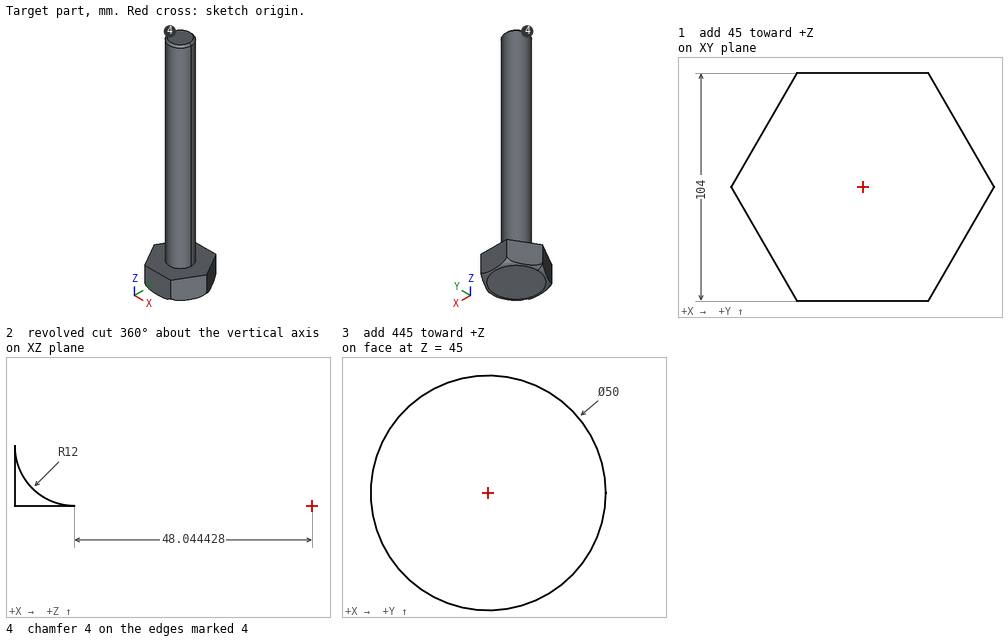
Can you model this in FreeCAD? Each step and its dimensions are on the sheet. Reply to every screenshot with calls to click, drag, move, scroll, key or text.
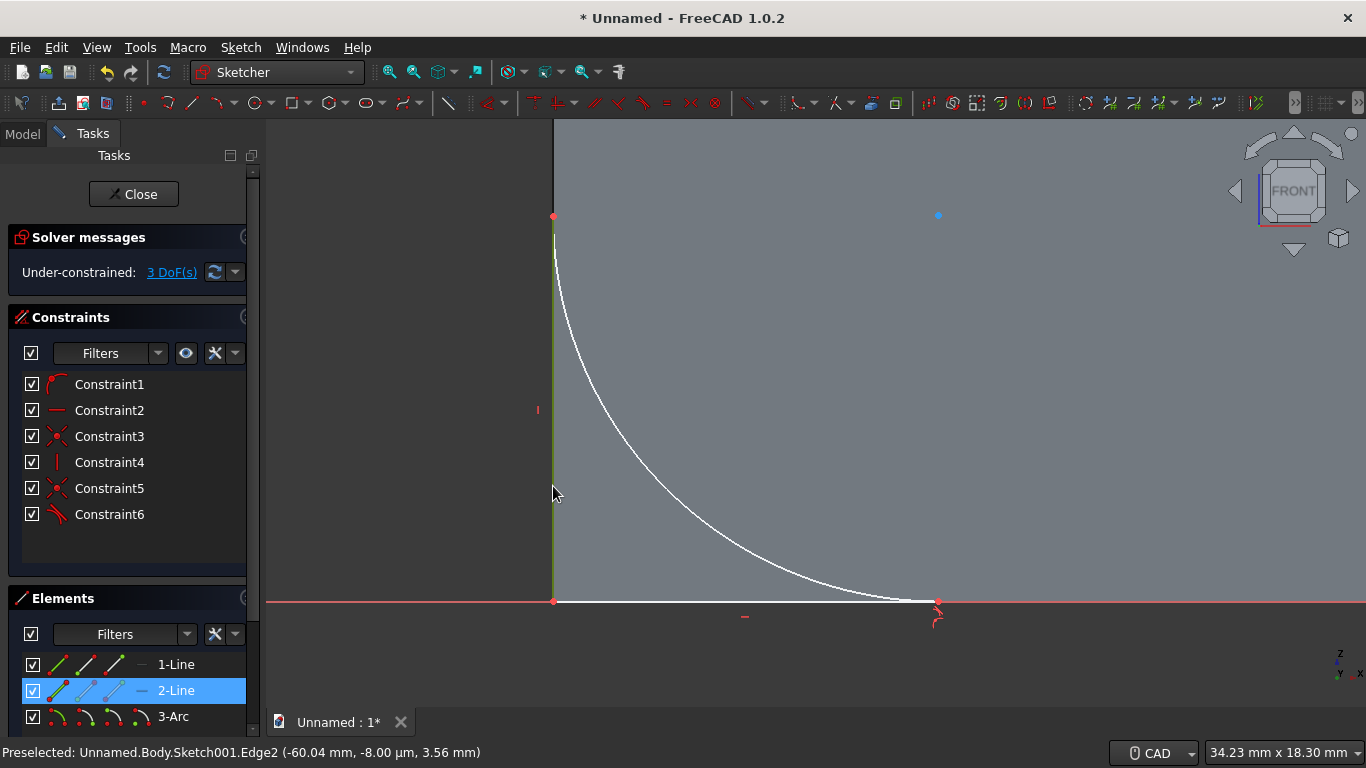
click(596, 392)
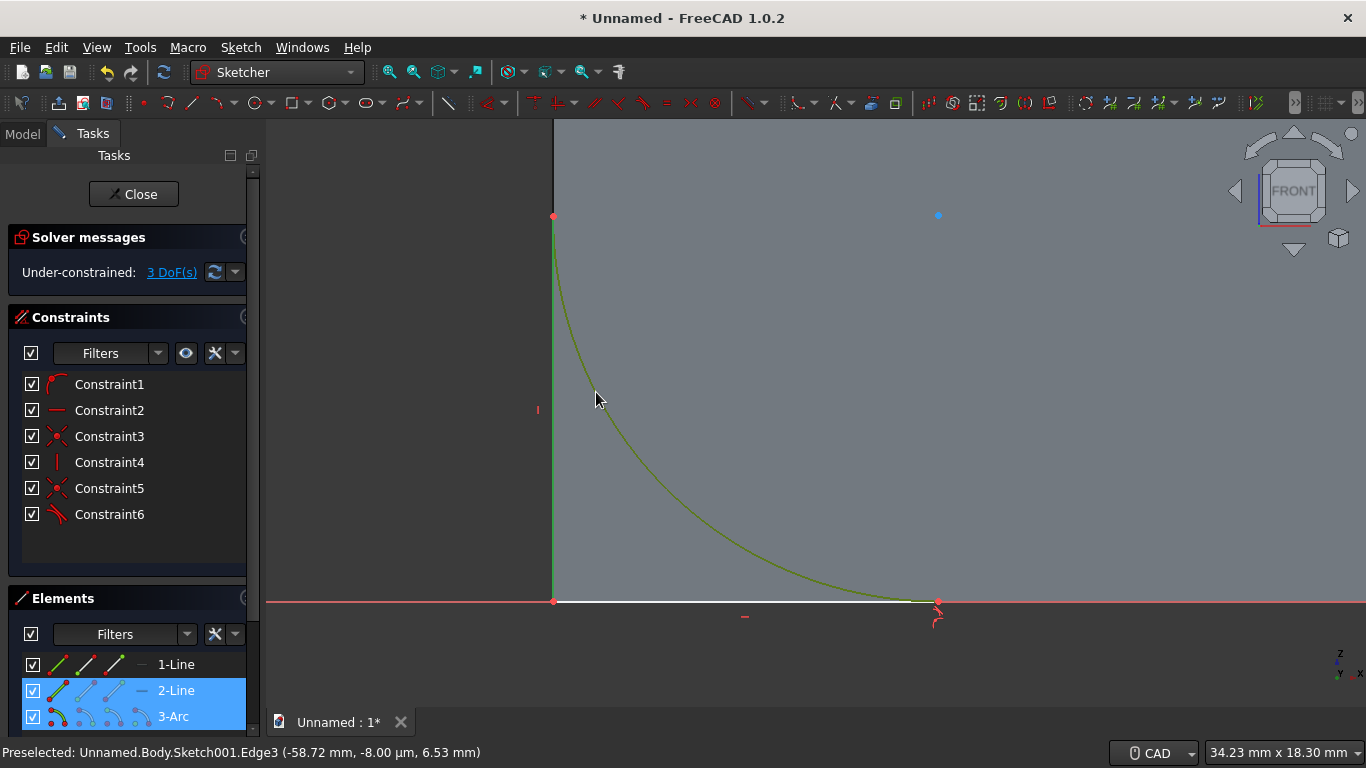
click(644, 104)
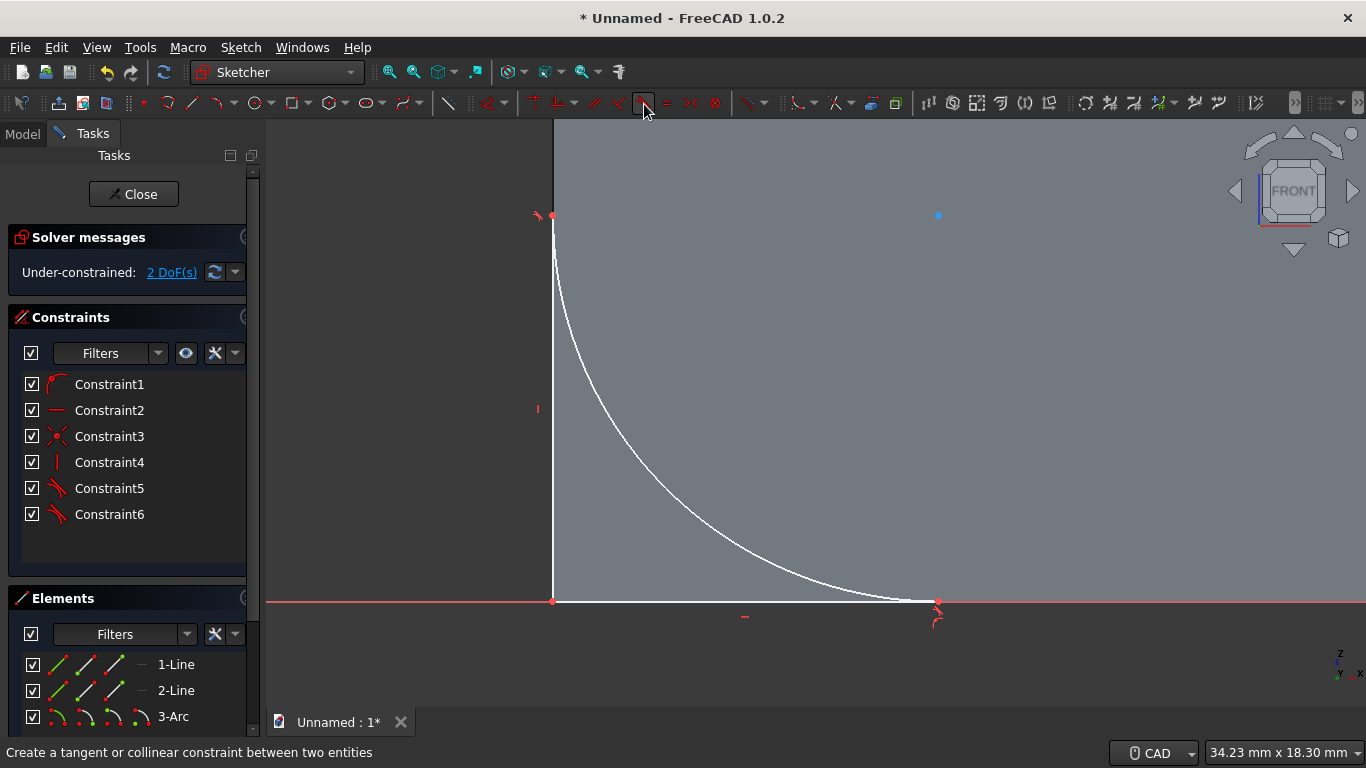
click(488, 104)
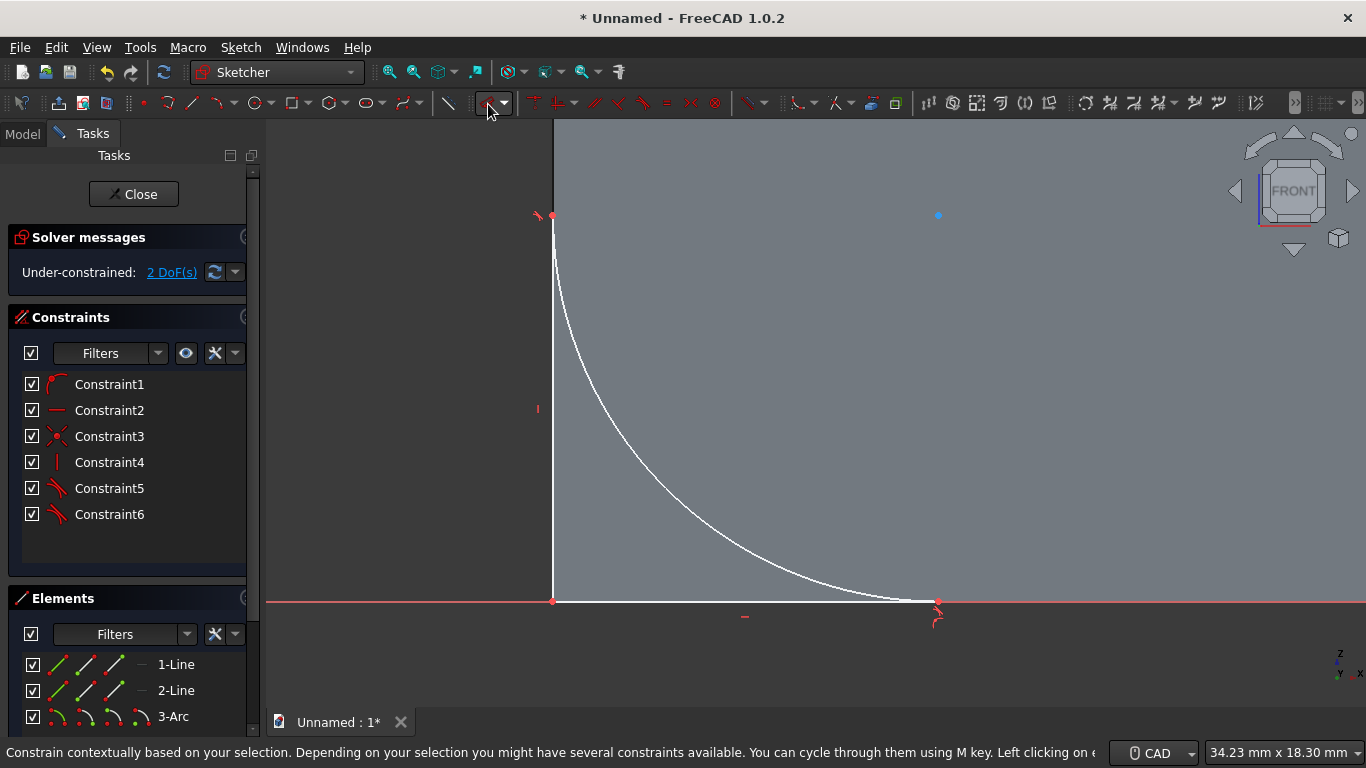
click(595, 391)
click(566, 406)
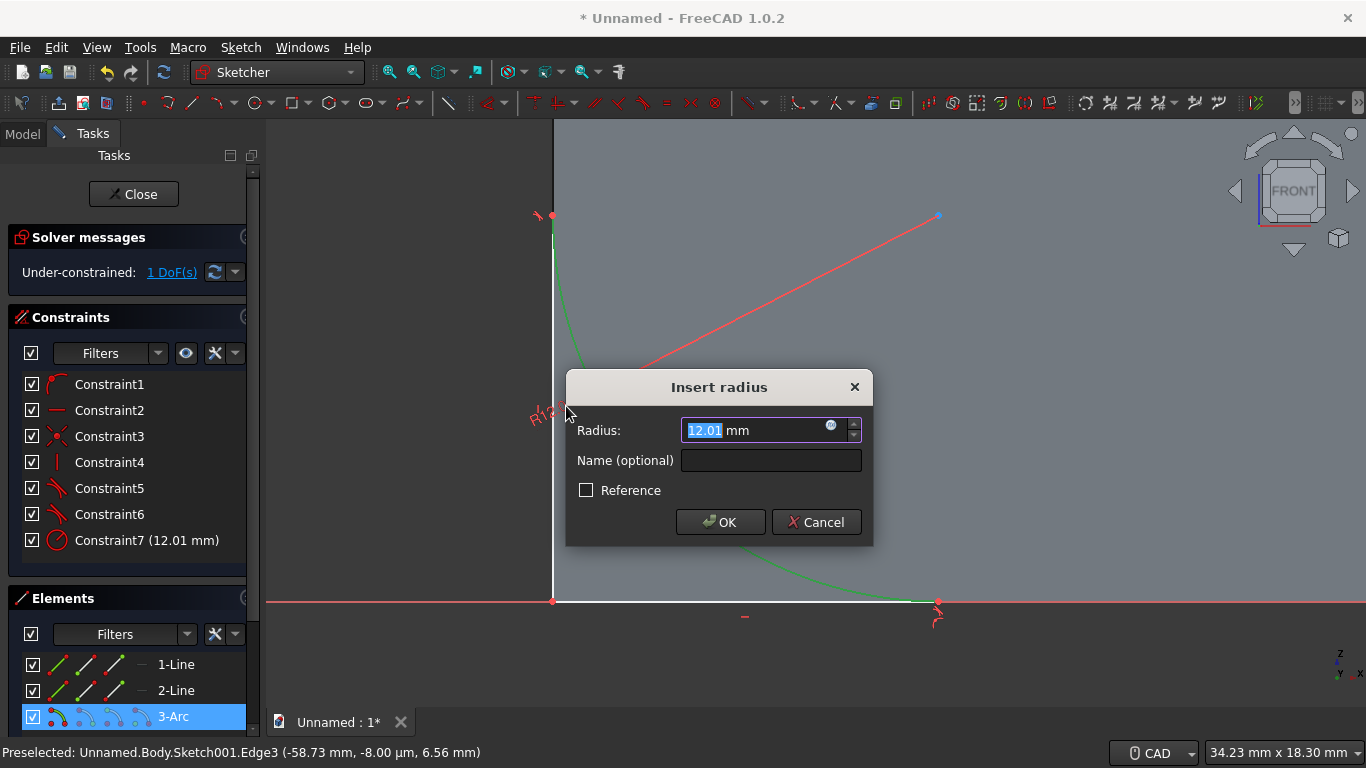
text(12)
key(Return)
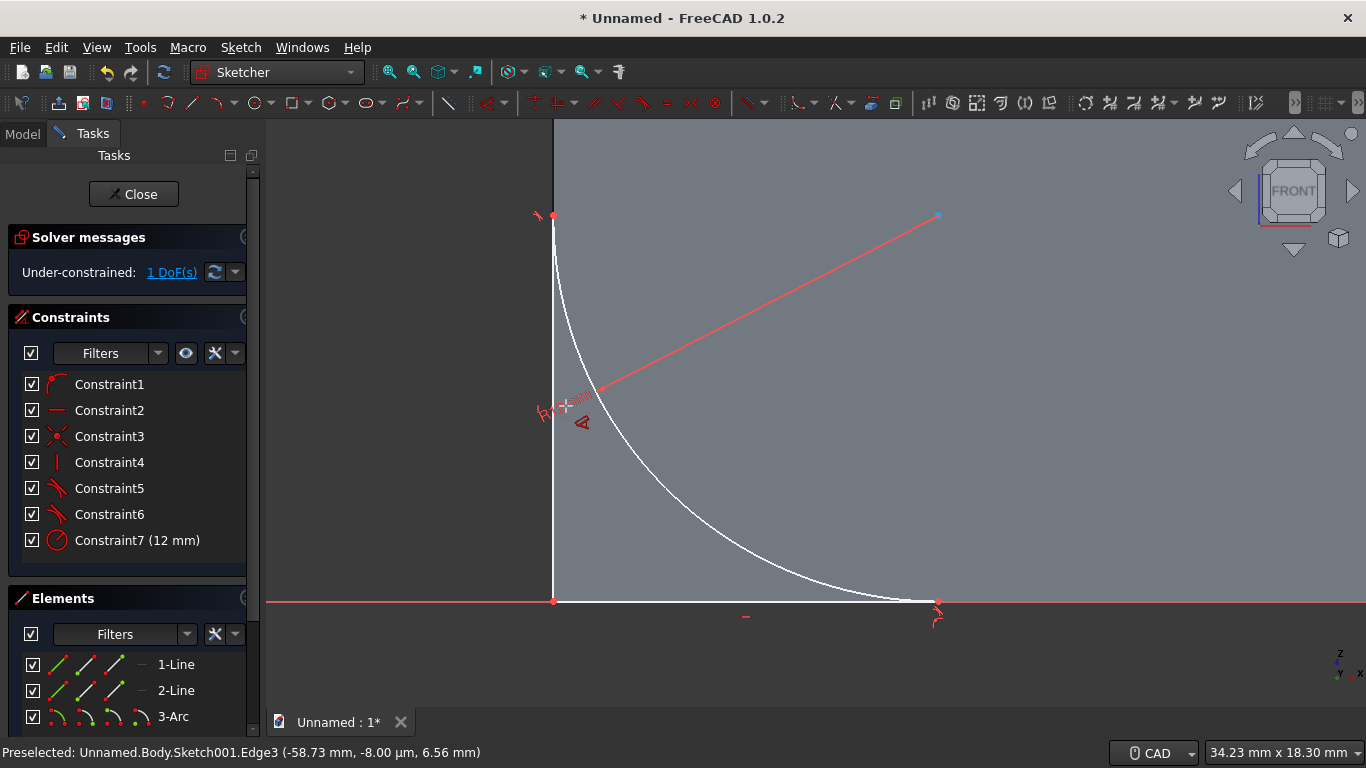
click(939, 602)
click(1070, 636)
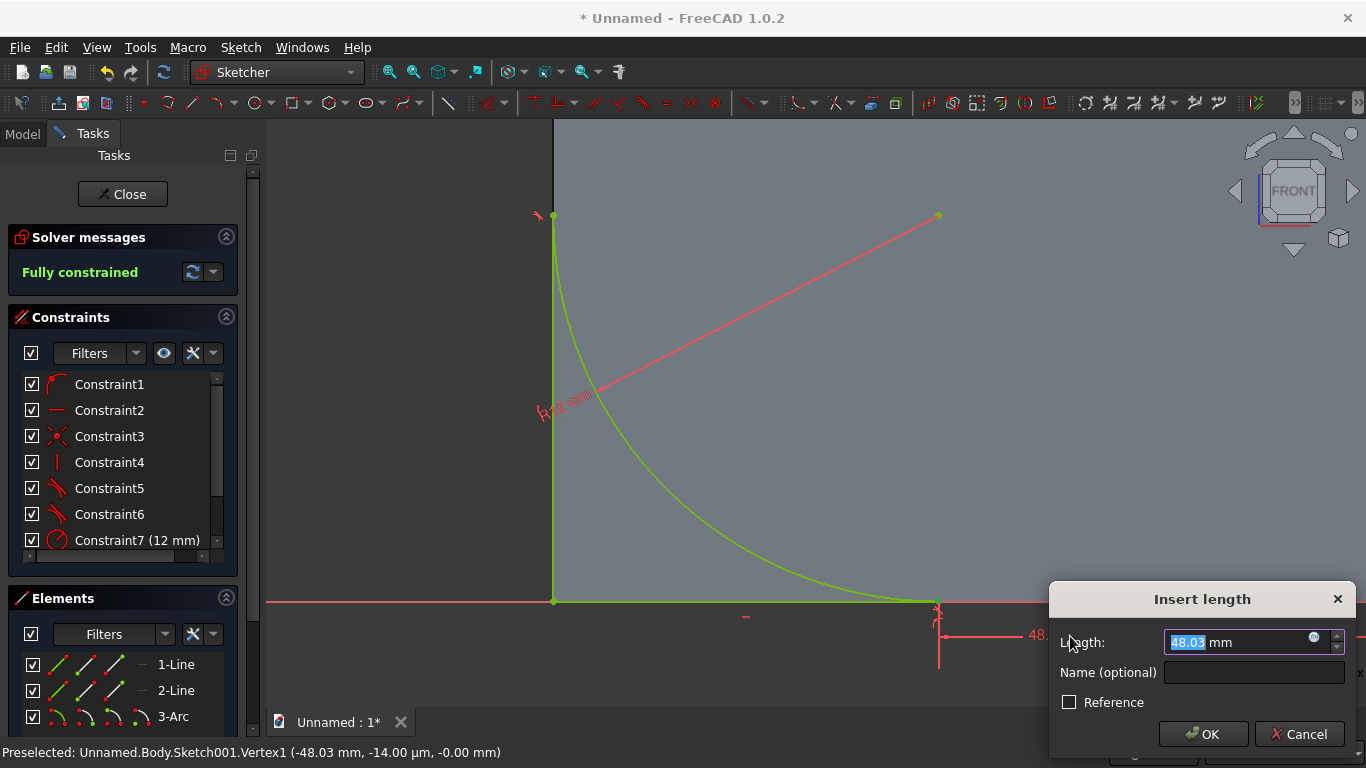
text(48.044428)
key(Return)
key(Escape)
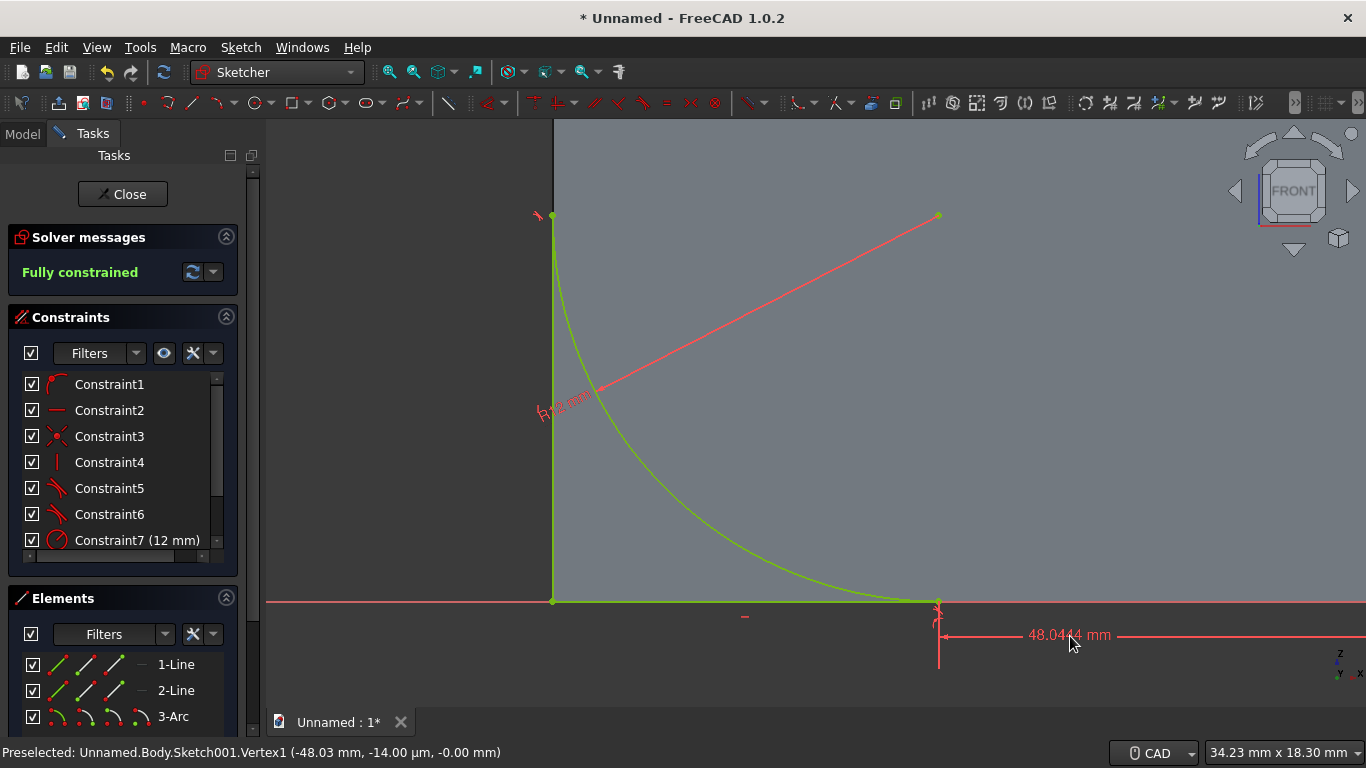
click(123, 194)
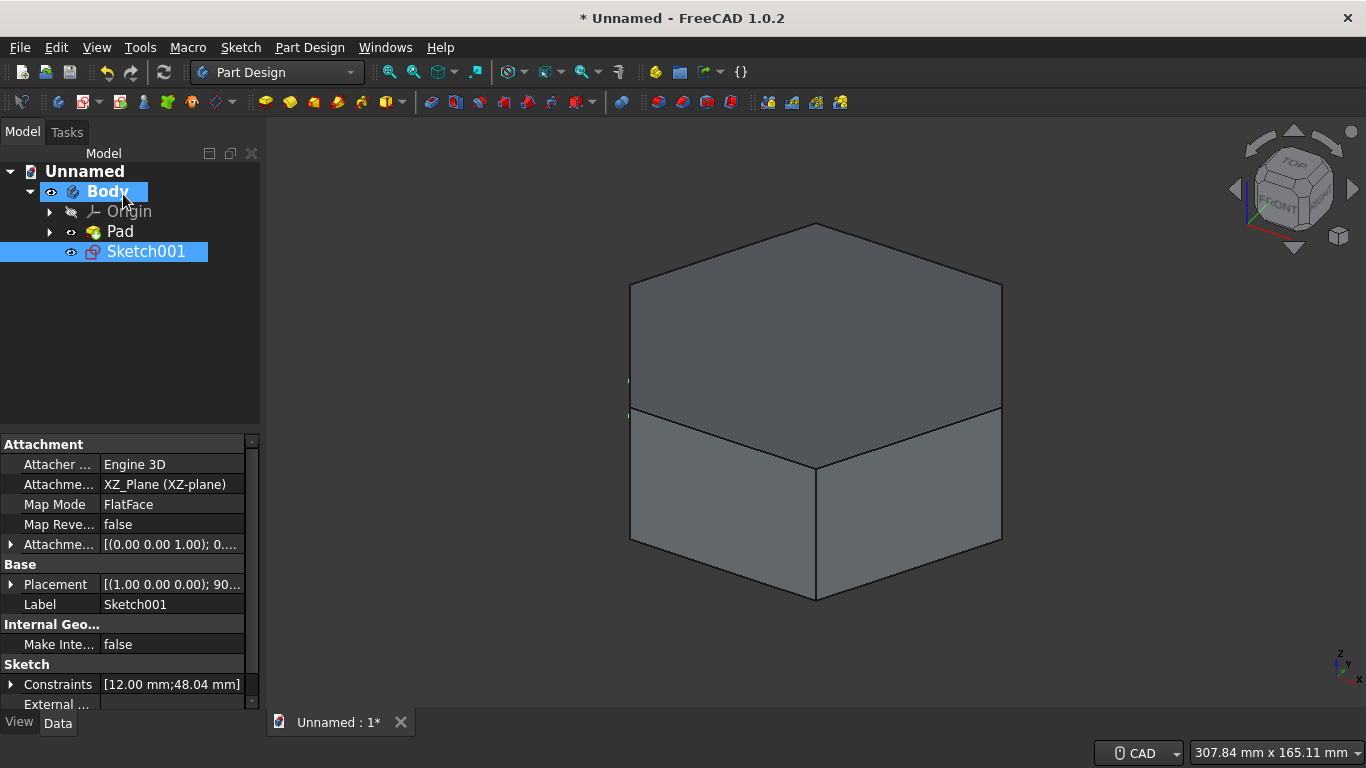
click(480, 102)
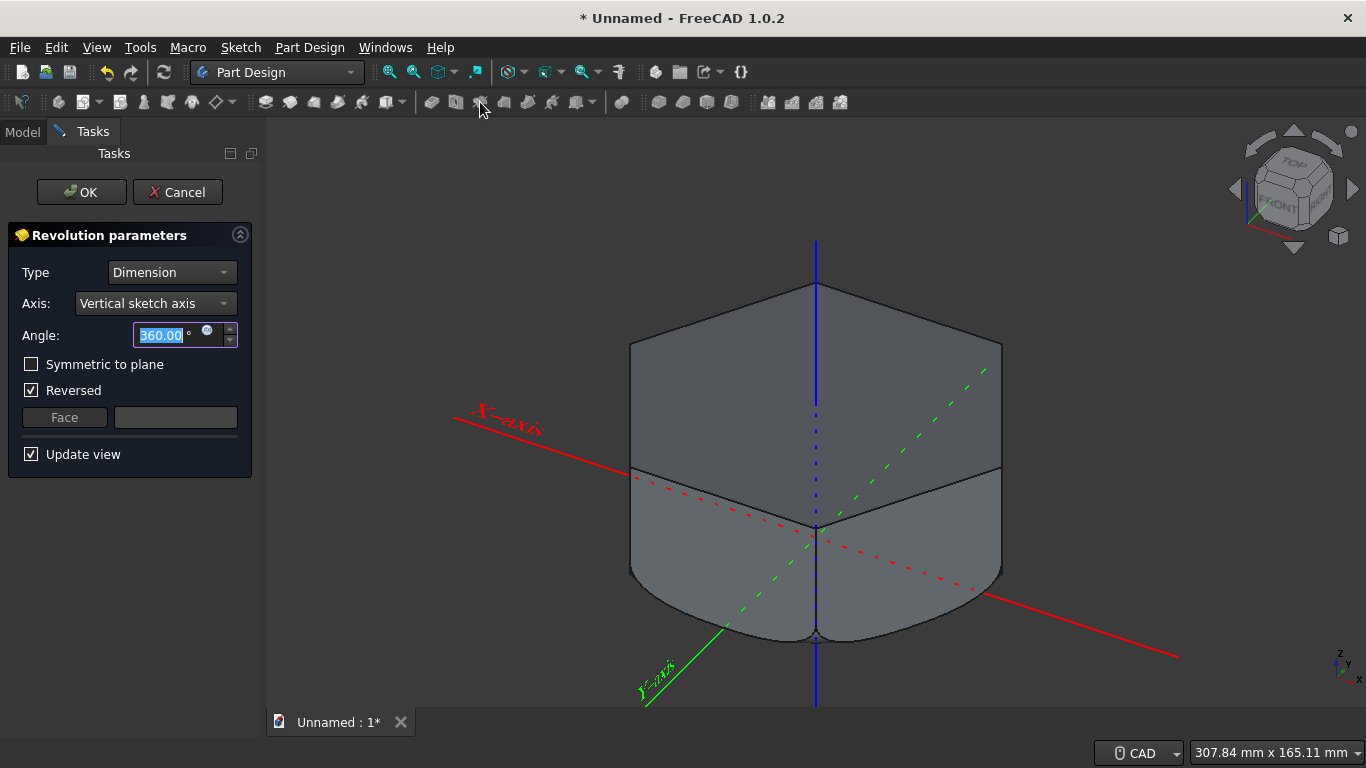
click(82, 192)